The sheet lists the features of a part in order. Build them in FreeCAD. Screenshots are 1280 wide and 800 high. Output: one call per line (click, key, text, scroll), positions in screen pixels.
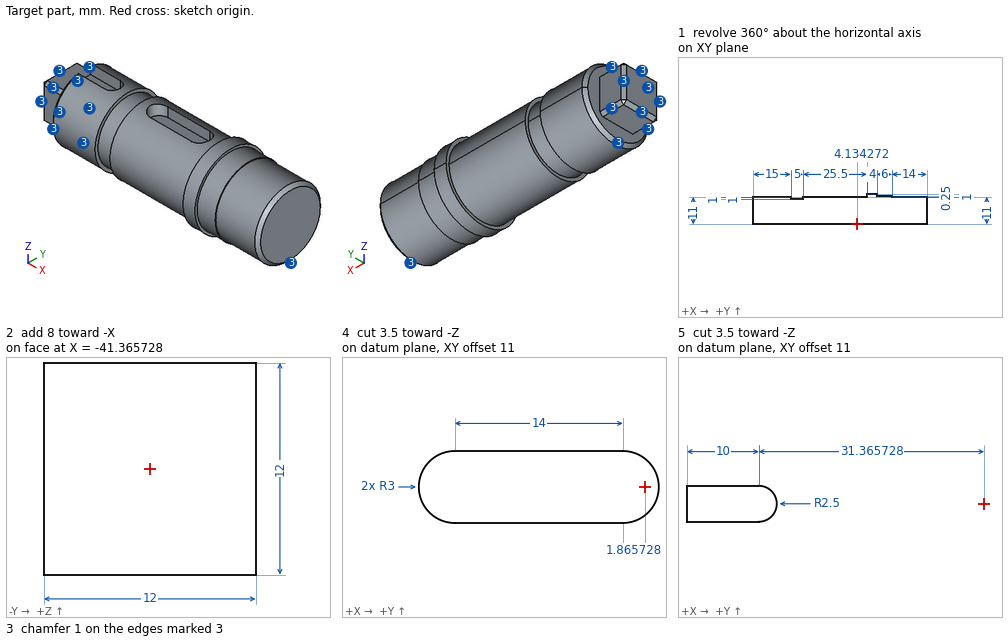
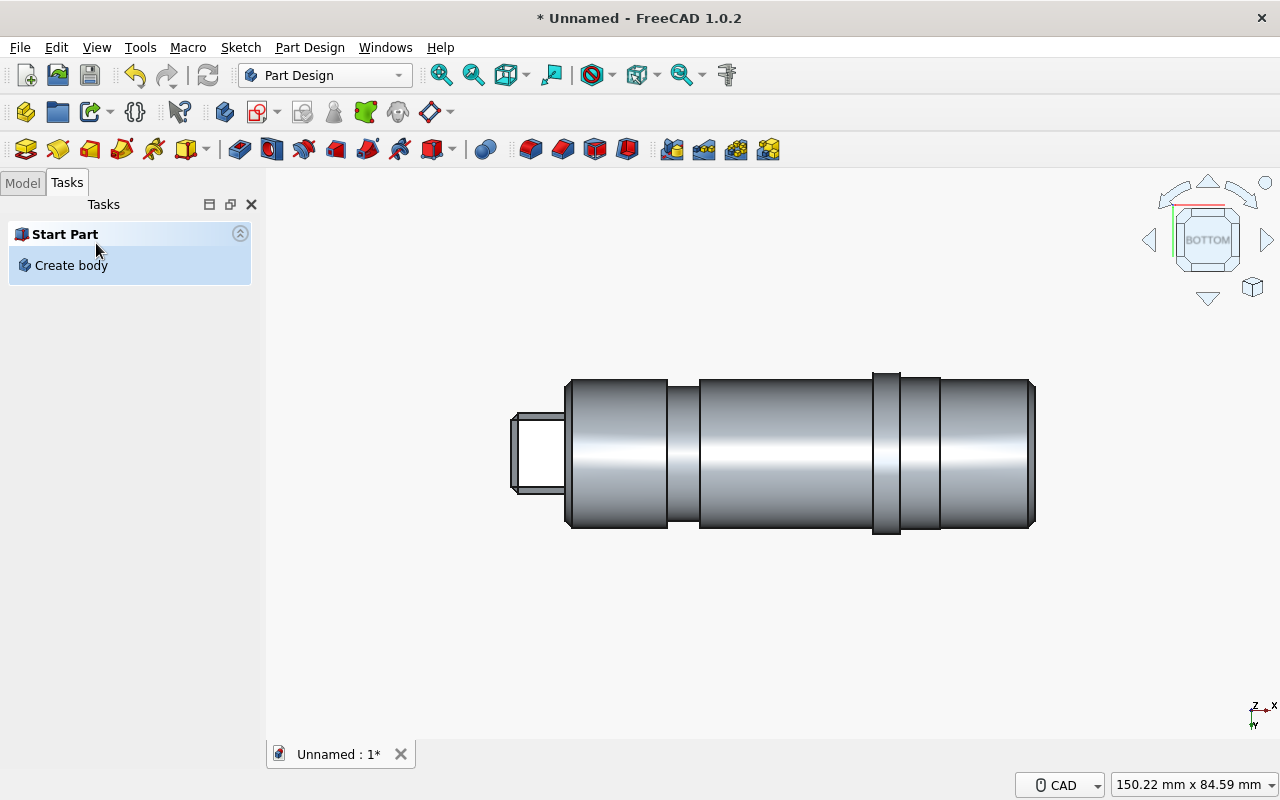
click(23, 182)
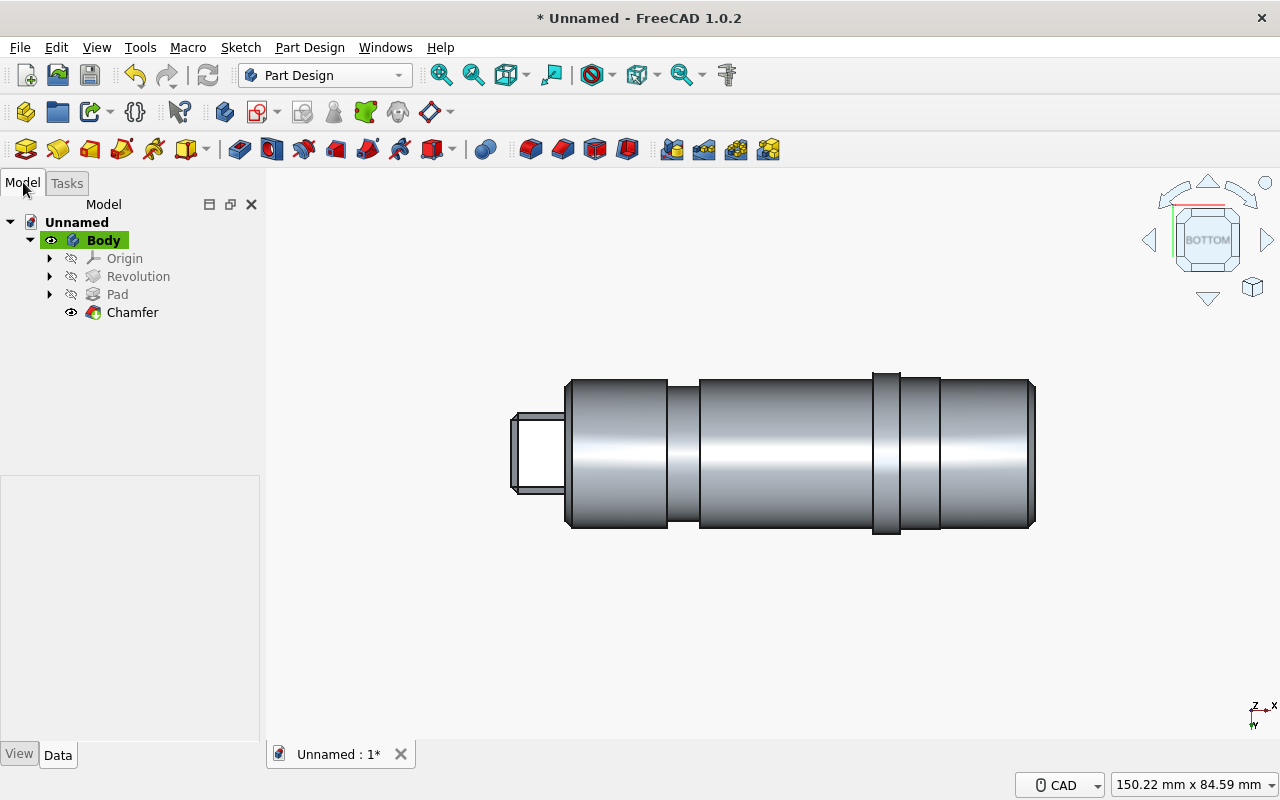
click(50, 258)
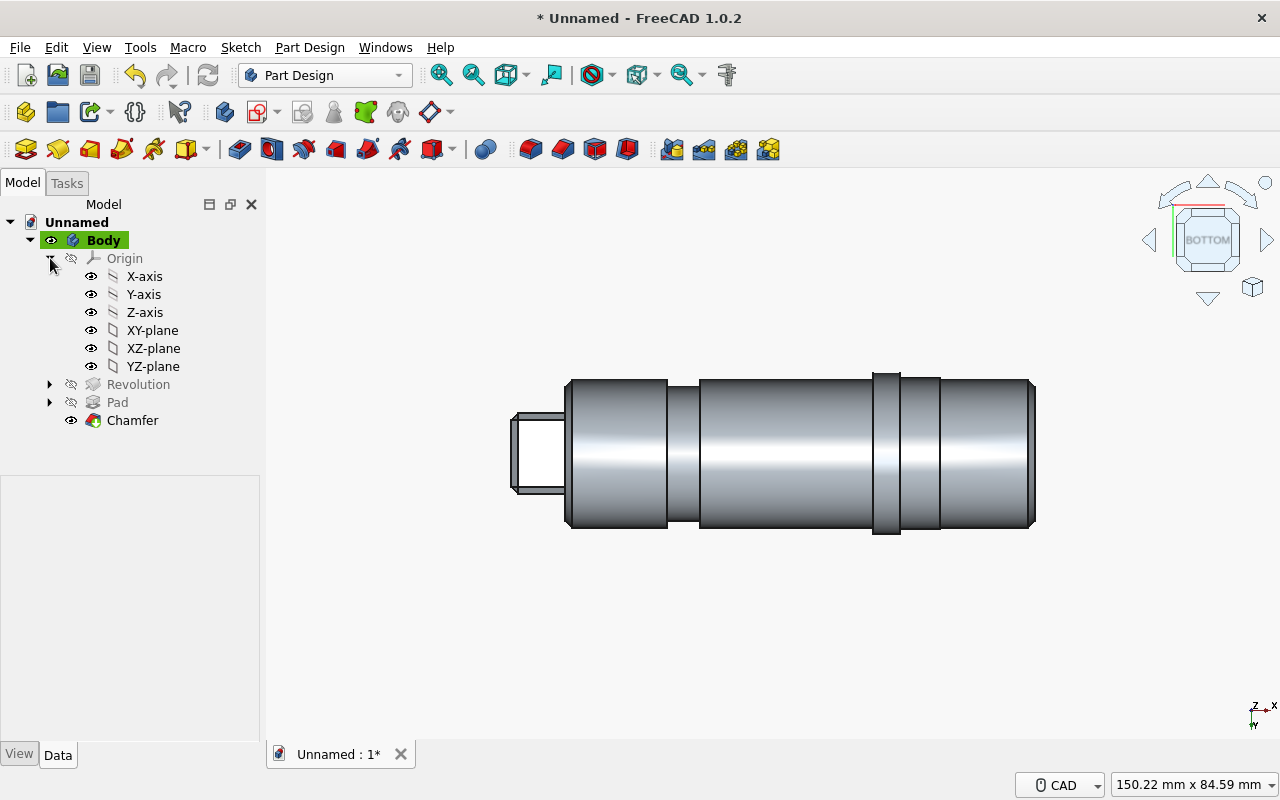
click(136, 330)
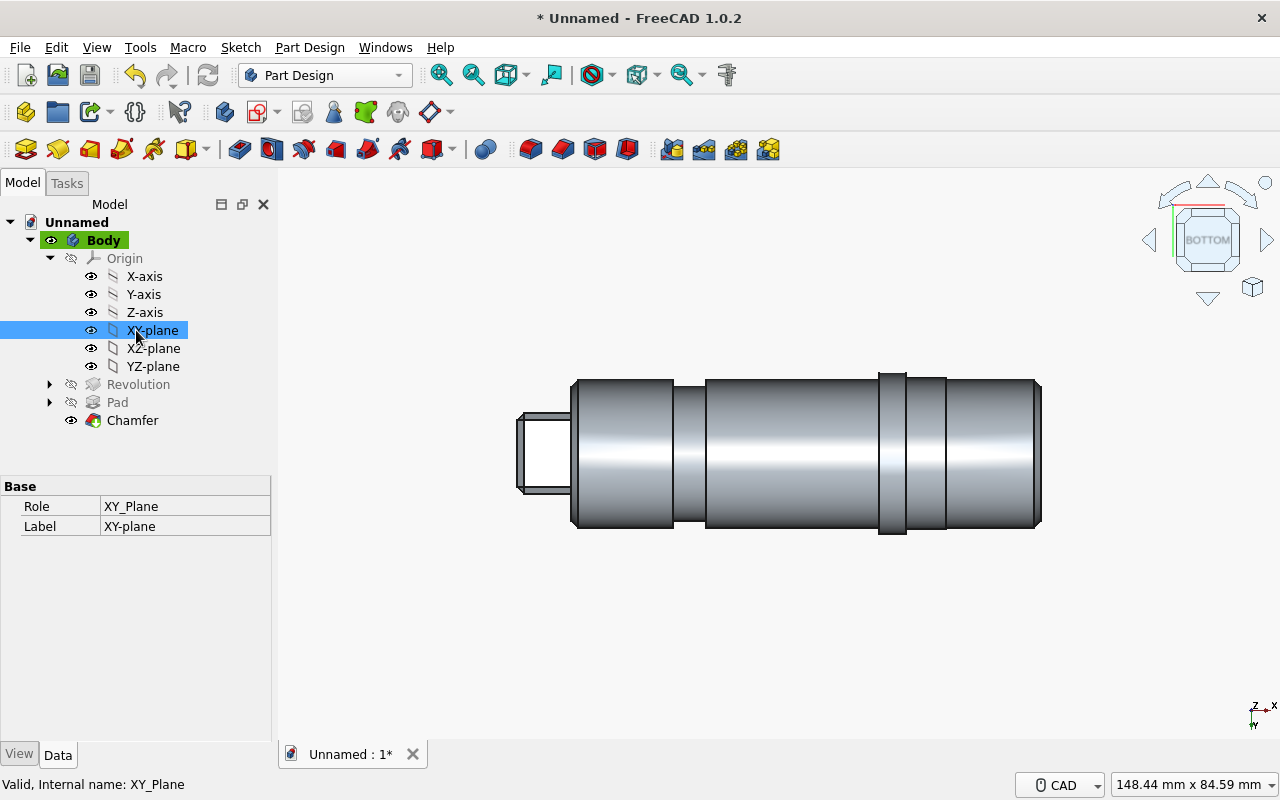
click(430, 112)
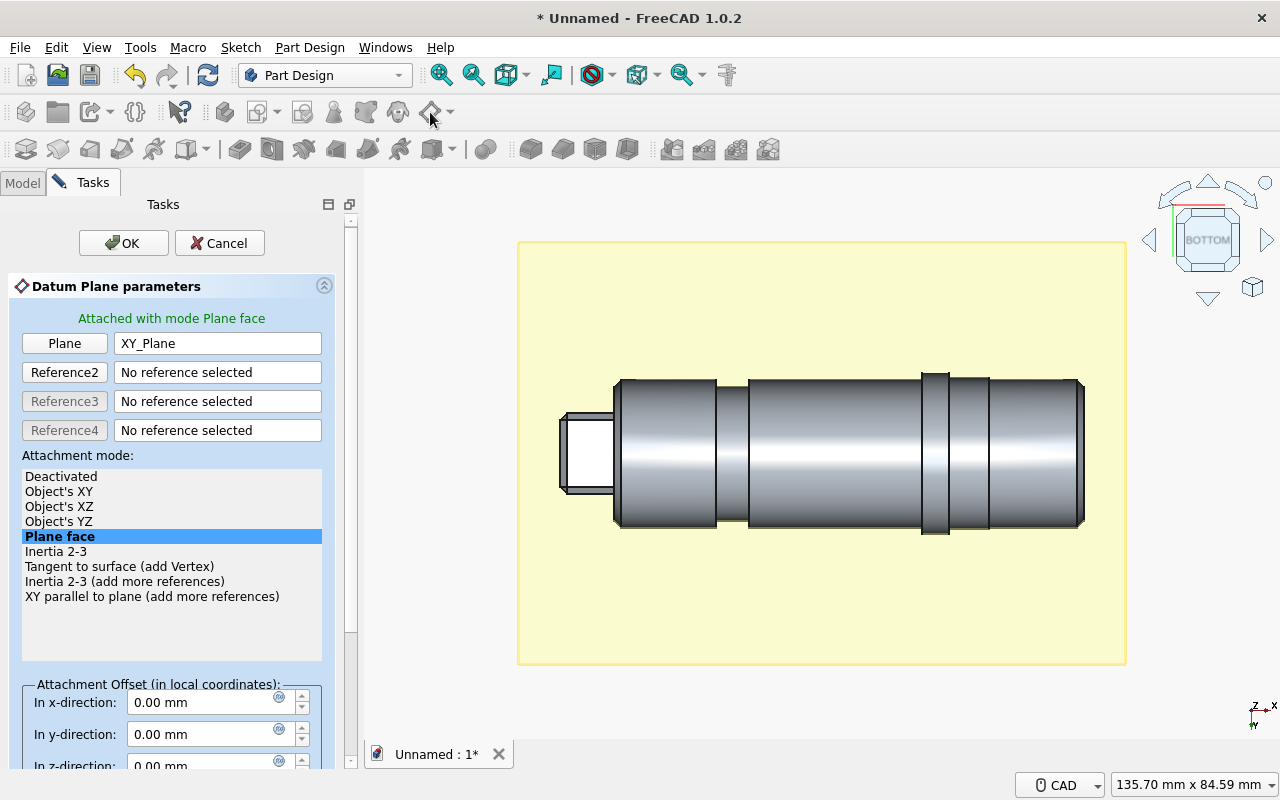
scroll(351, 491, down, 2)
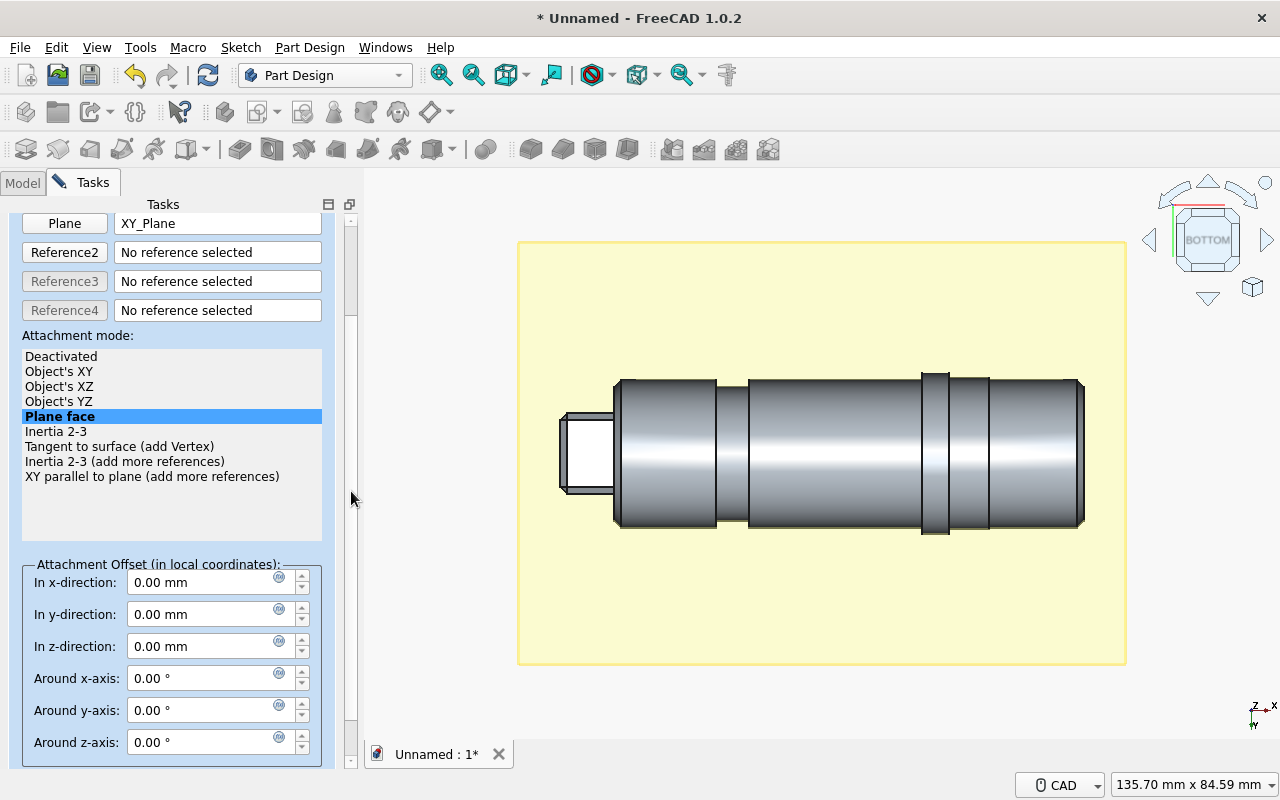
triple_click(210, 646)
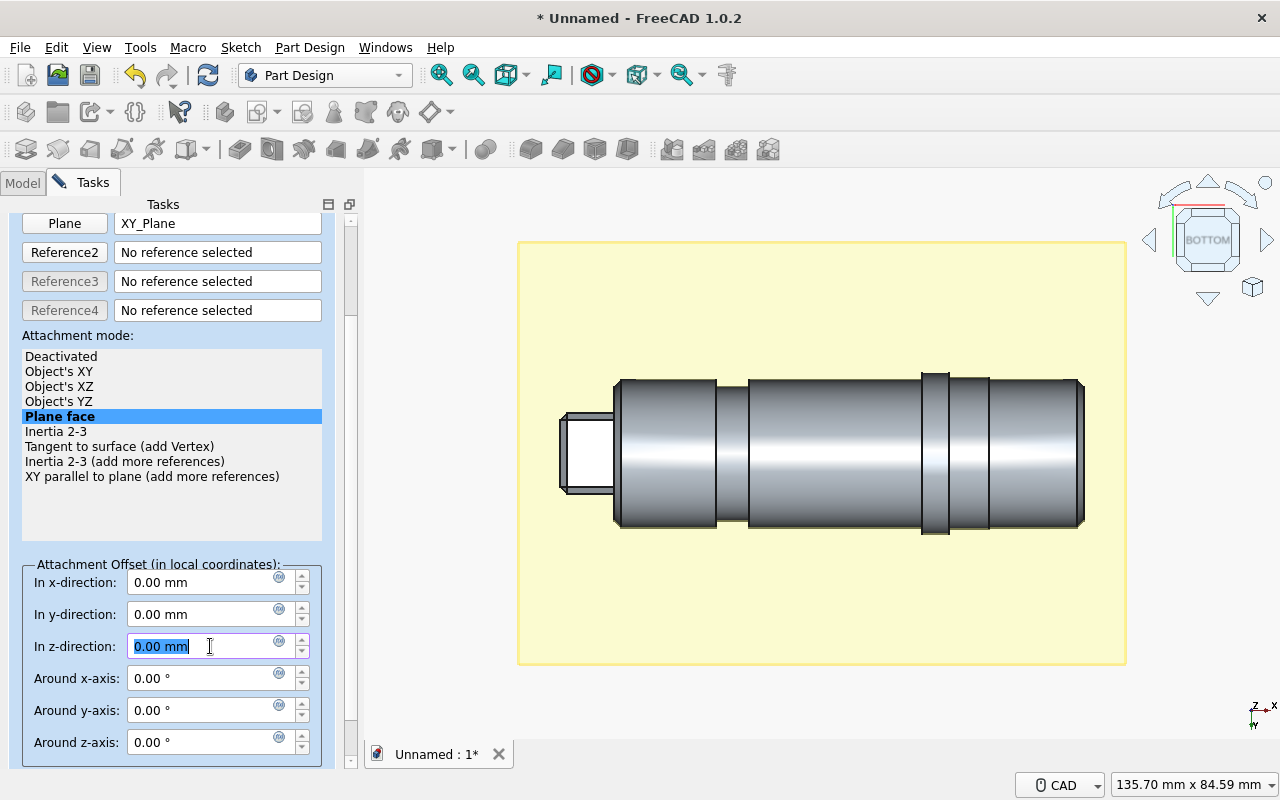
text(11)
key(Tab)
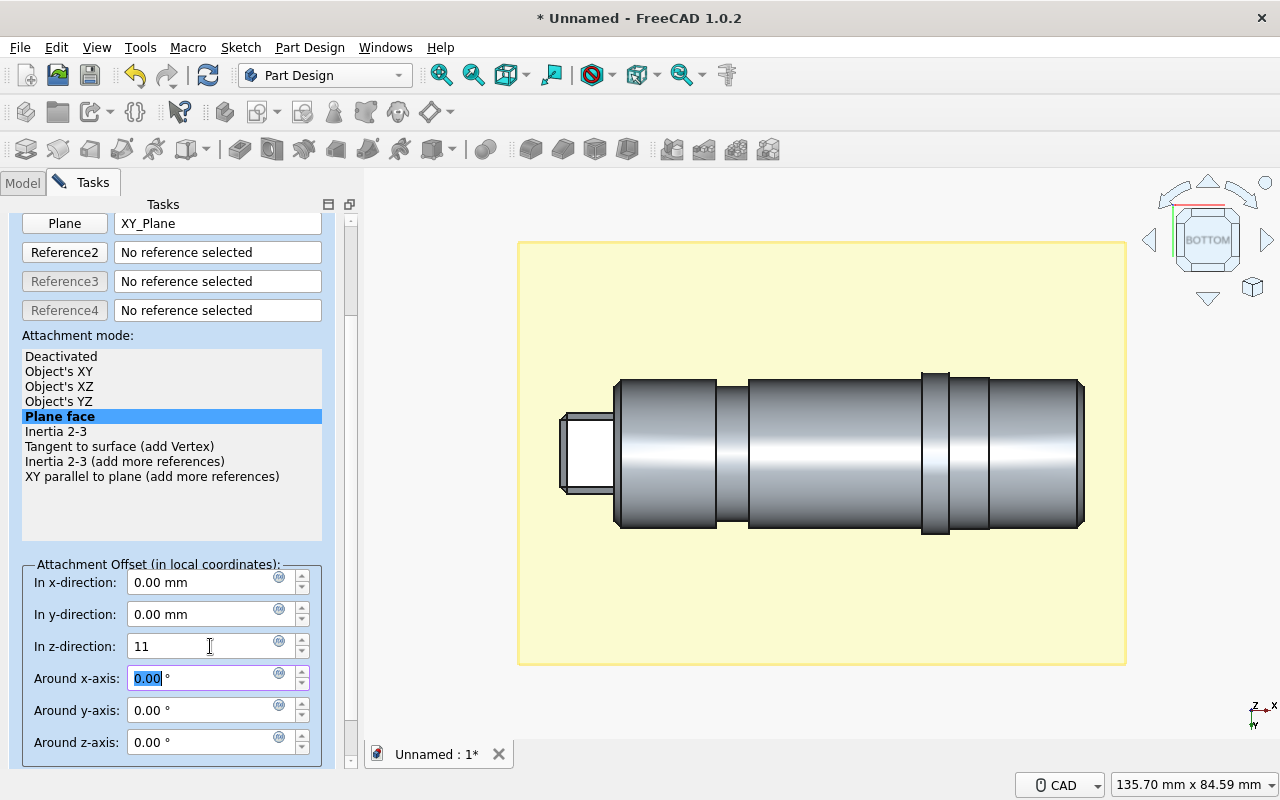
scroll(351, 491, up, 3)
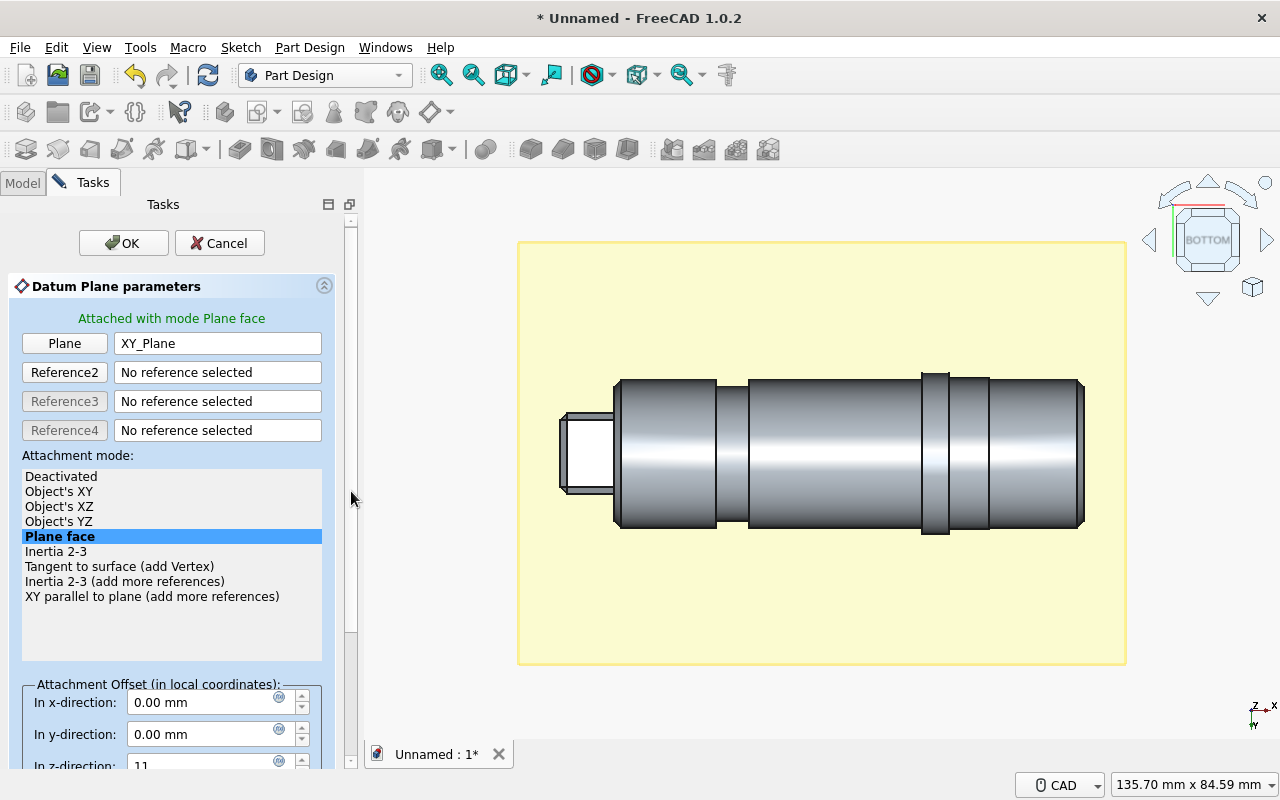
click(124, 243)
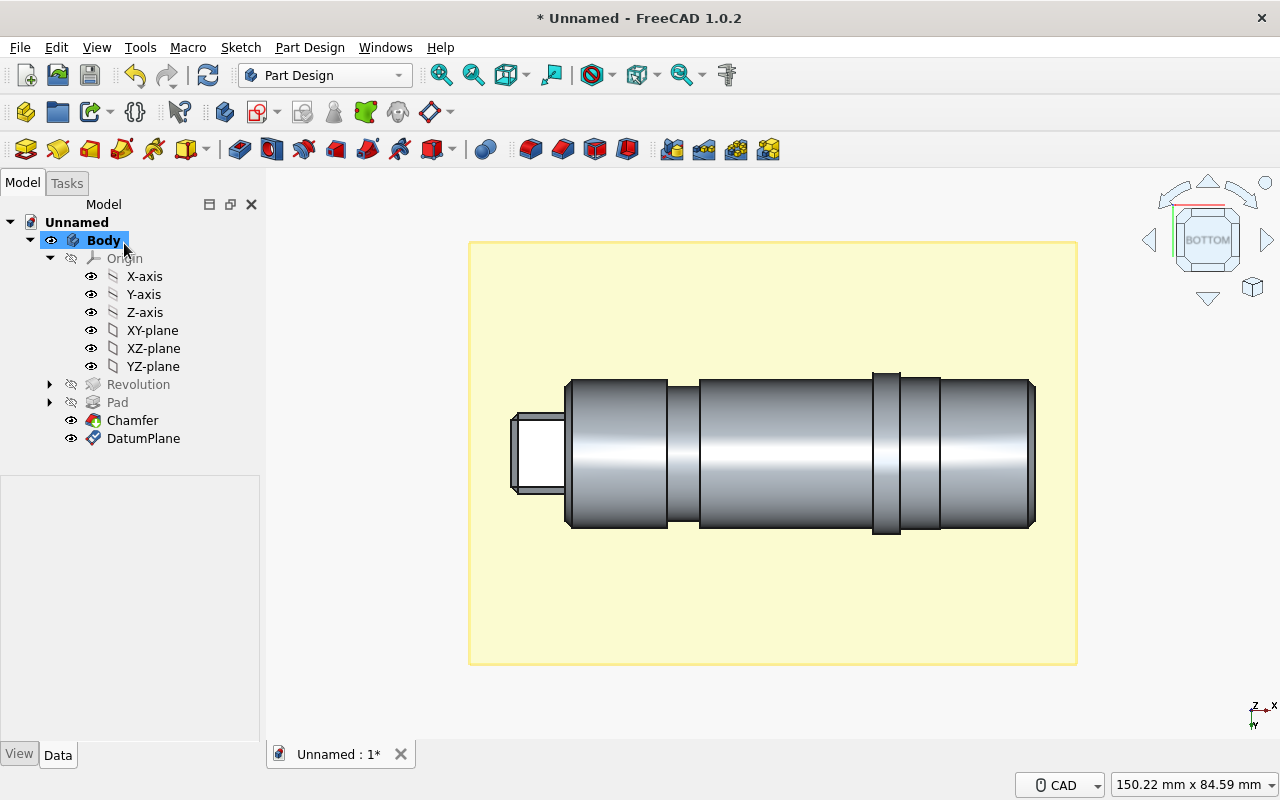
click(116, 438)